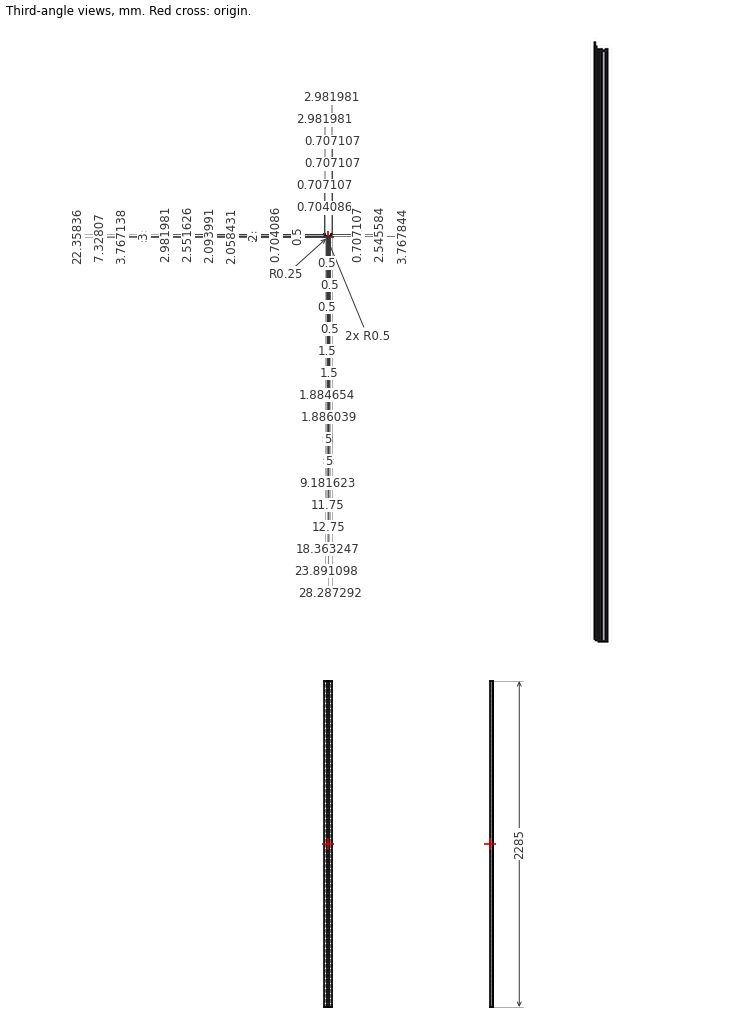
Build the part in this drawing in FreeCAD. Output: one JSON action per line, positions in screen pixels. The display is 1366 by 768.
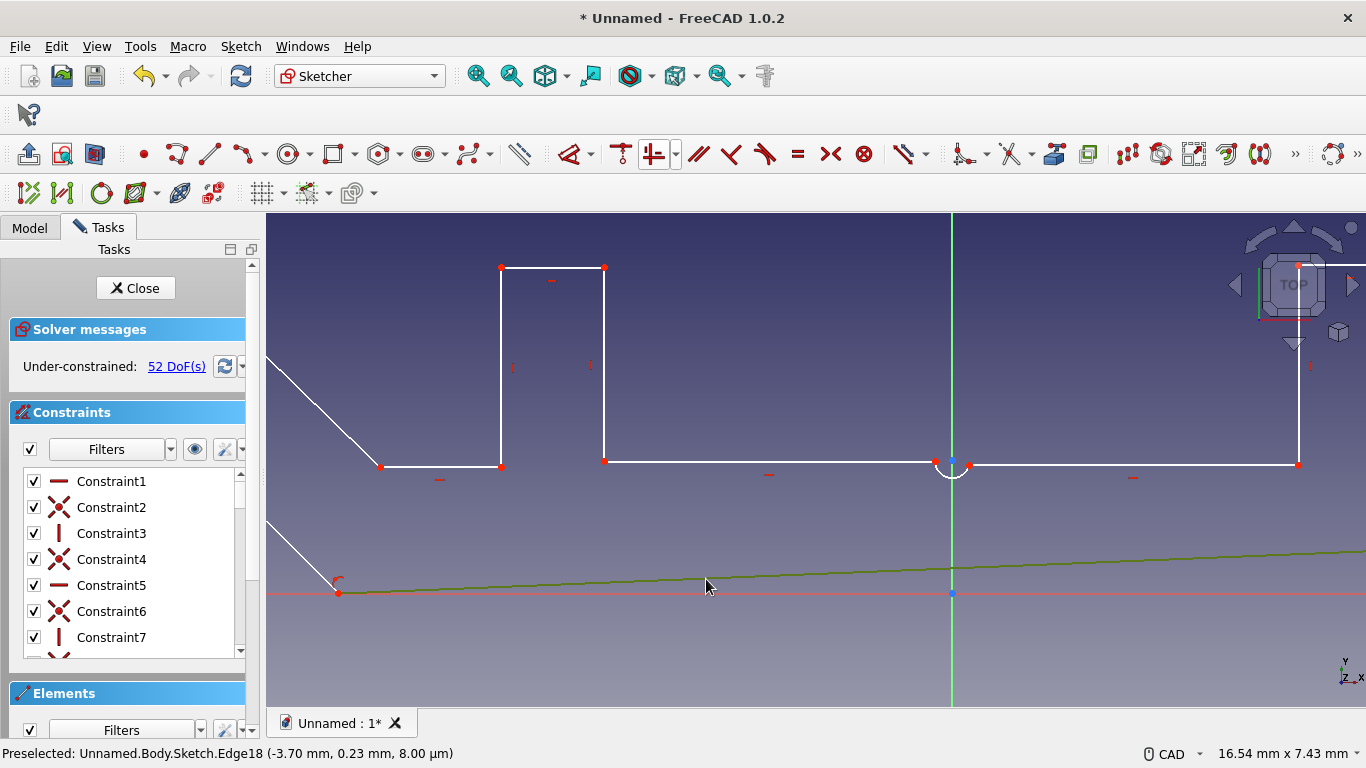
{"action": "key", "text": "h"}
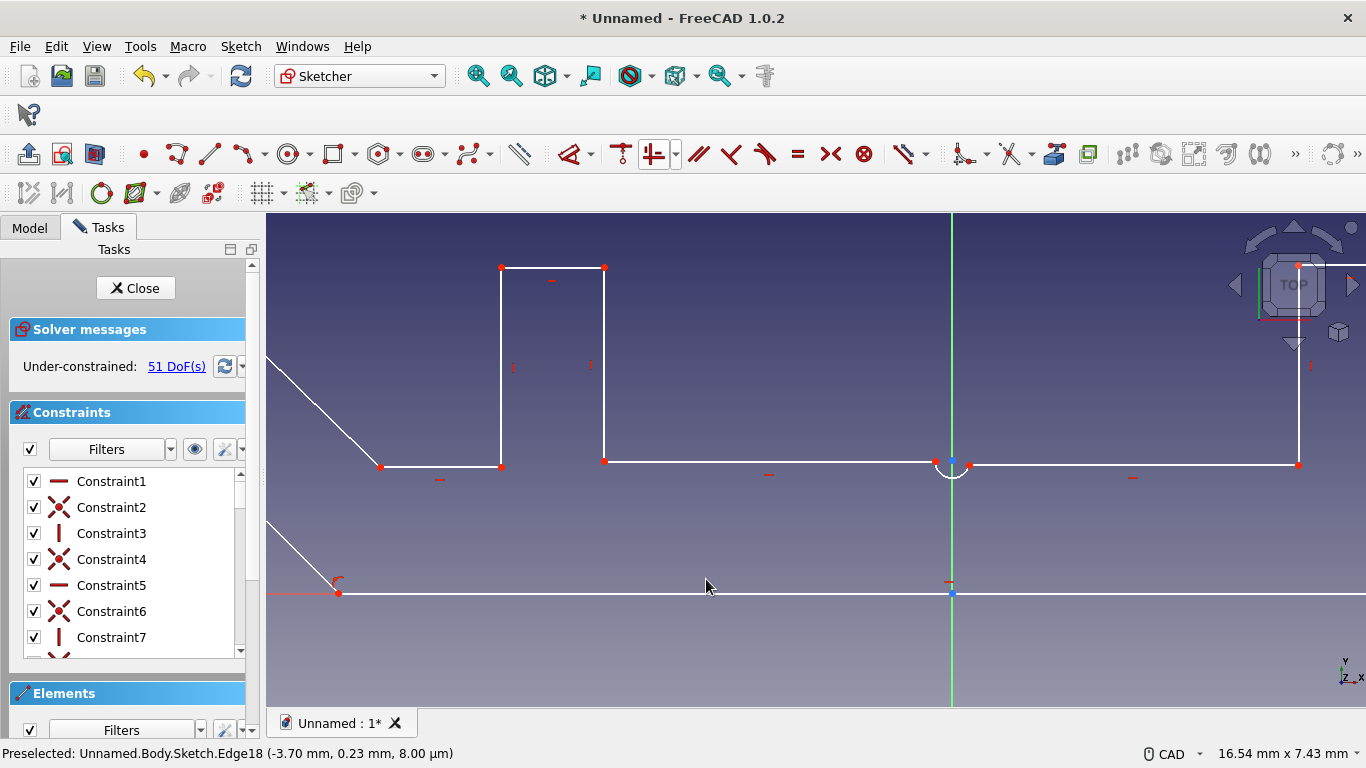
{"action": "scroll", "coordinate": [707, 581], "scroll_direction": "down", "scroll_amount": 9}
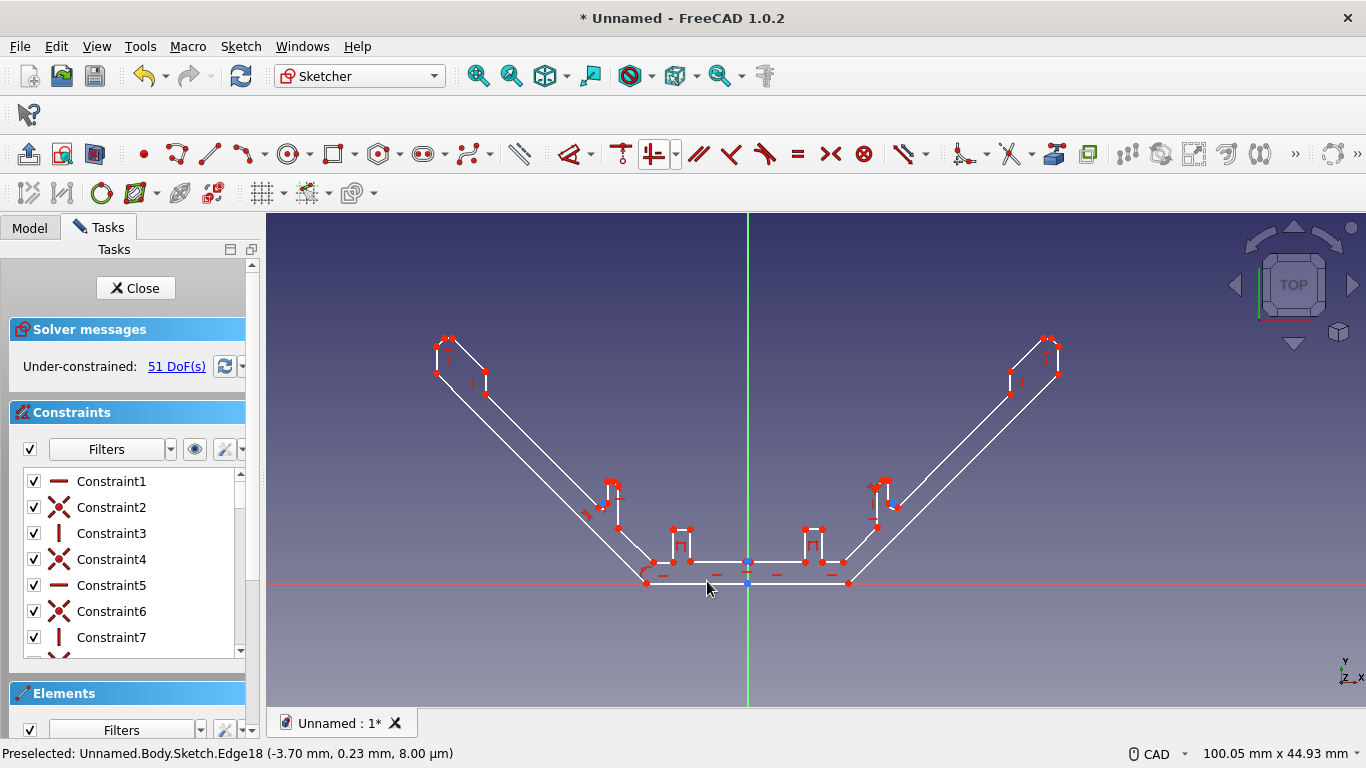
{"action": "scroll", "coordinate": [602, 509], "scroll_direction": "up", "scroll_amount": 7}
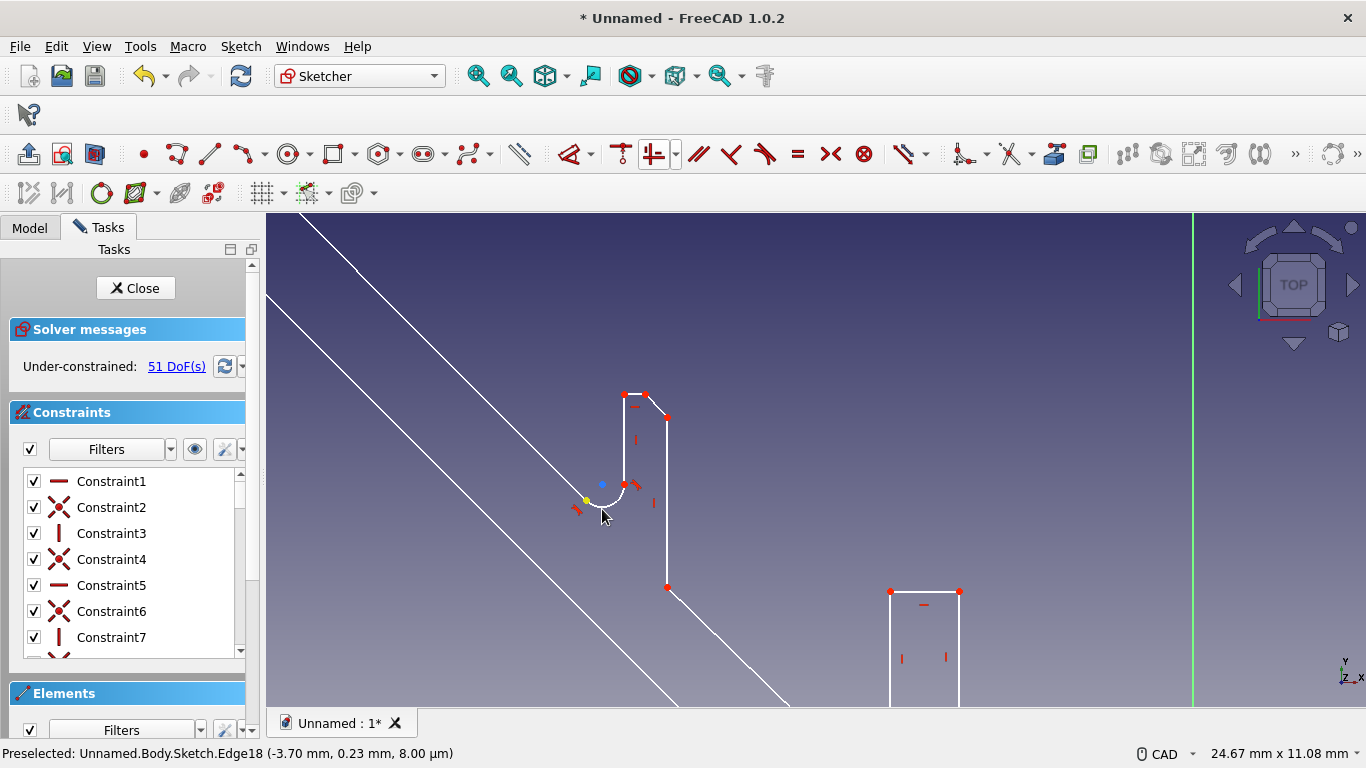
{"action": "left_click", "coordinate": [600, 507]}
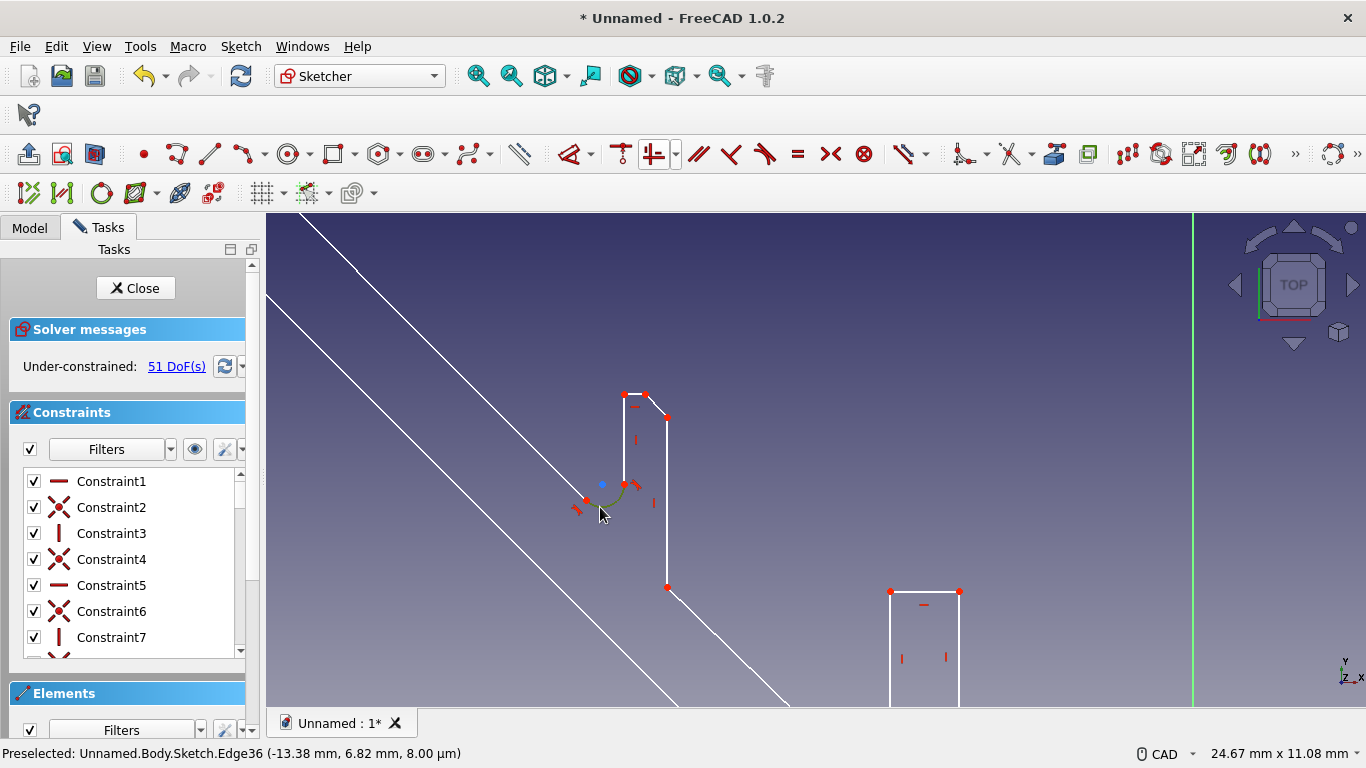
{"action": "scroll", "coordinate": [602, 509], "scroll_direction": "down", "scroll_amount": 7}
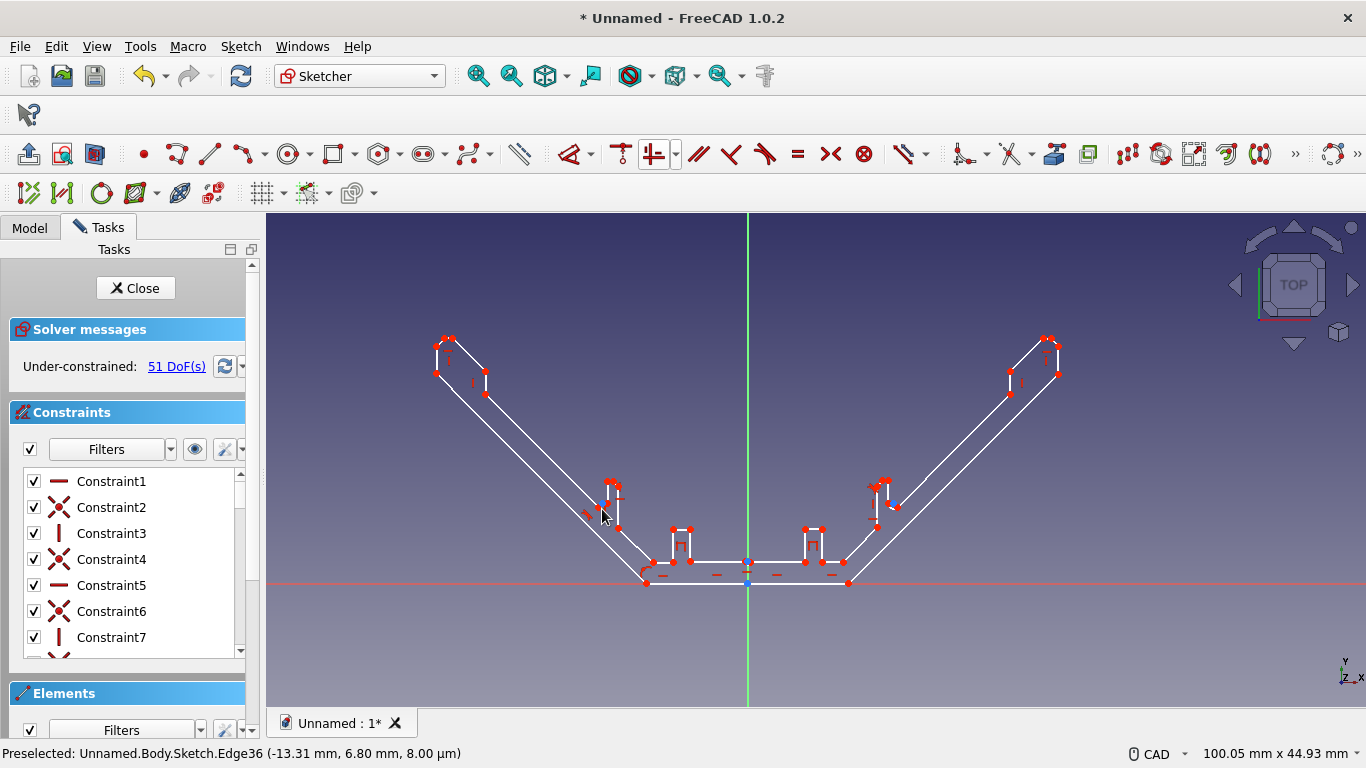
{"action": "scroll", "coordinate": [889, 507], "scroll_direction": "up", "scroll_amount": 7}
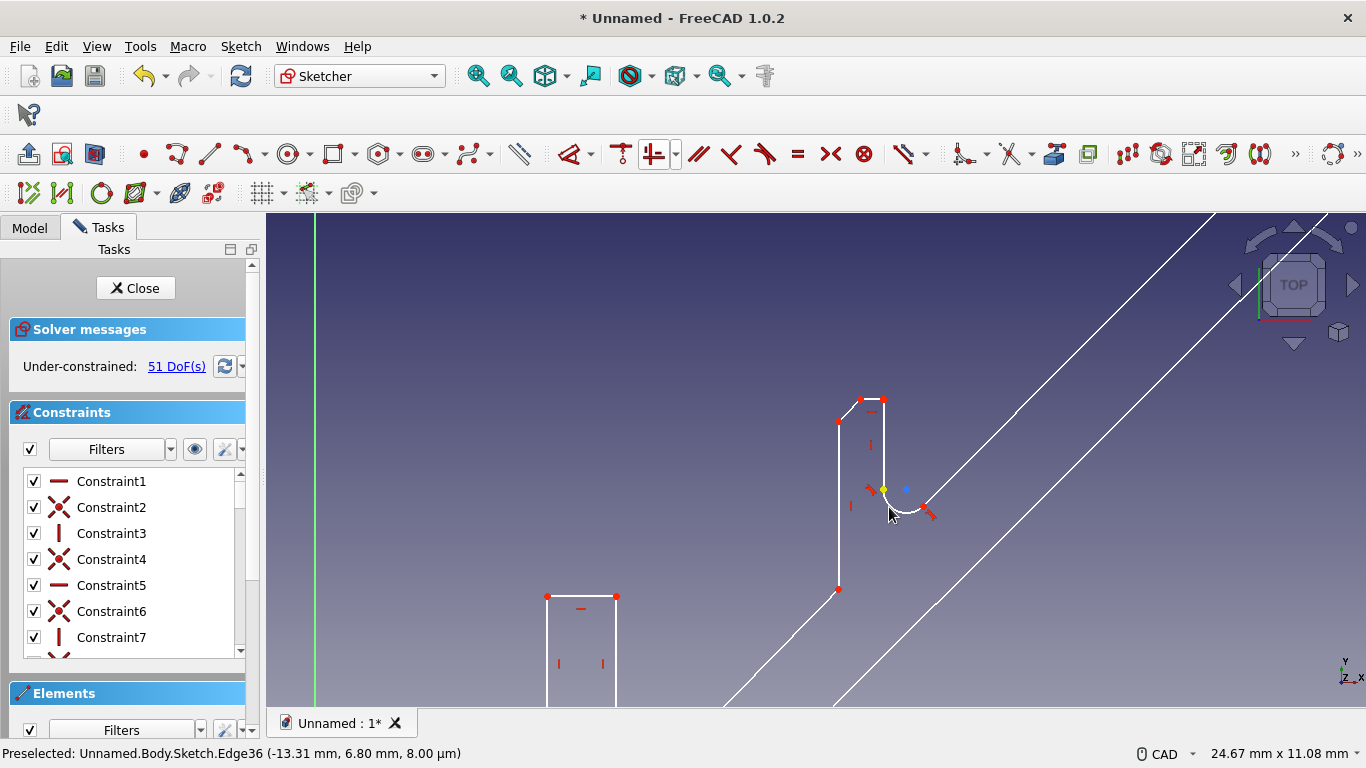
{"action": "left_click", "coordinate": [889, 505]}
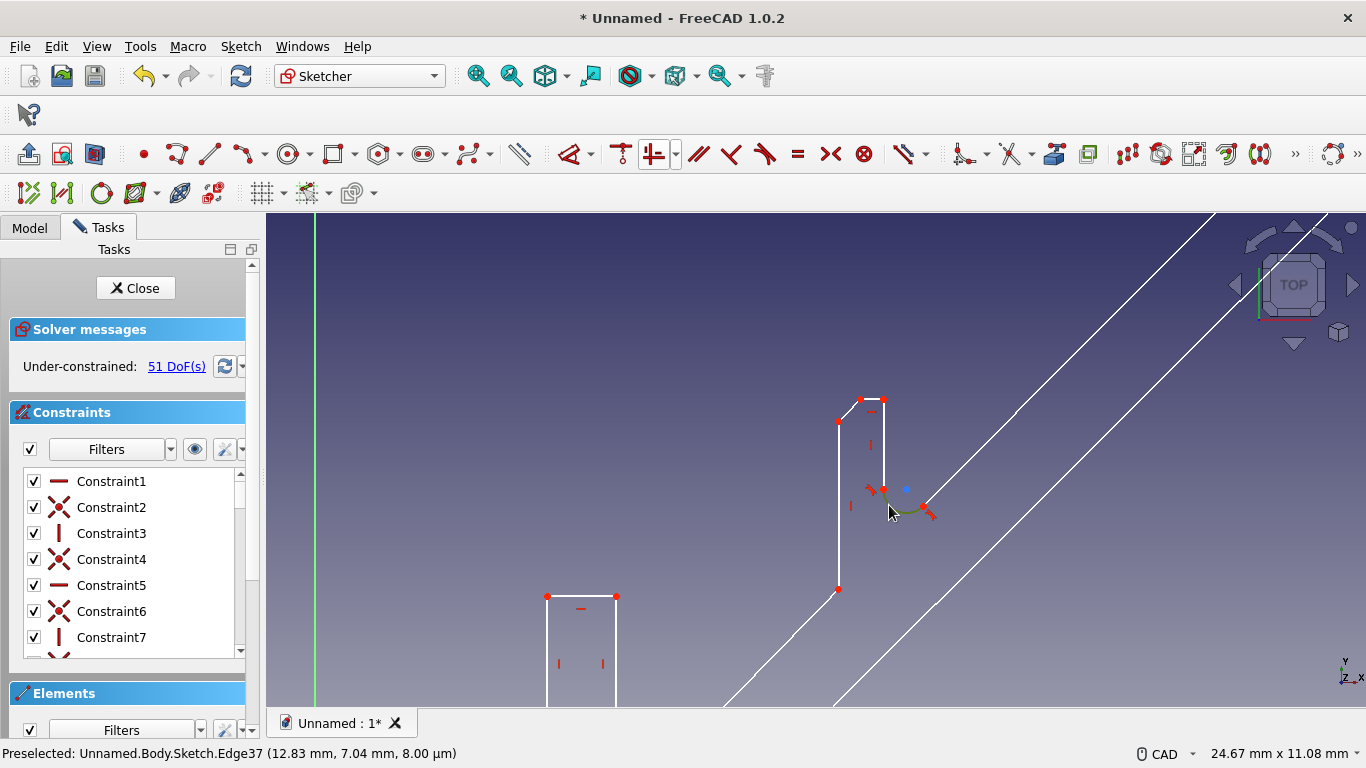
{"action": "left_click", "coordinate": [798, 154]}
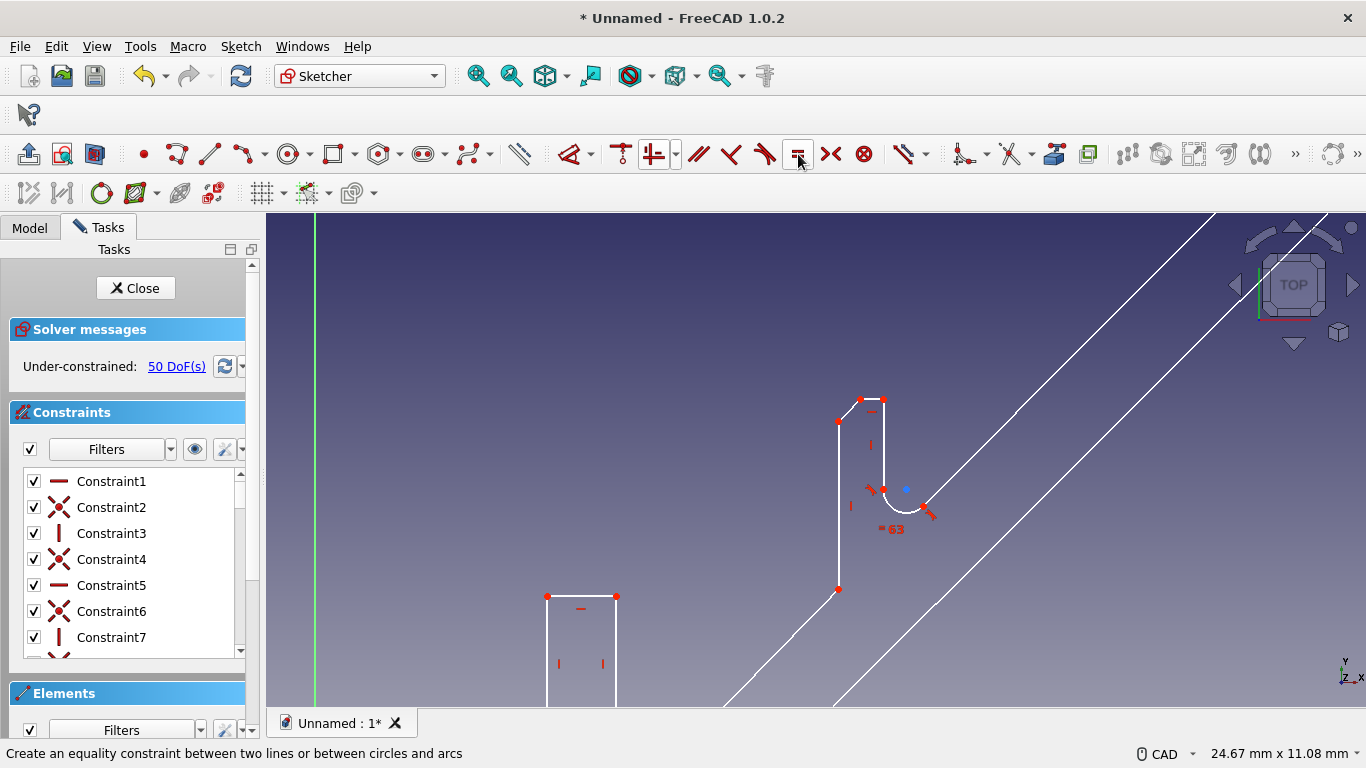
{"action": "scroll", "coordinate": [889, 507], "scroll_direction": "down", "scroll_amount": 7}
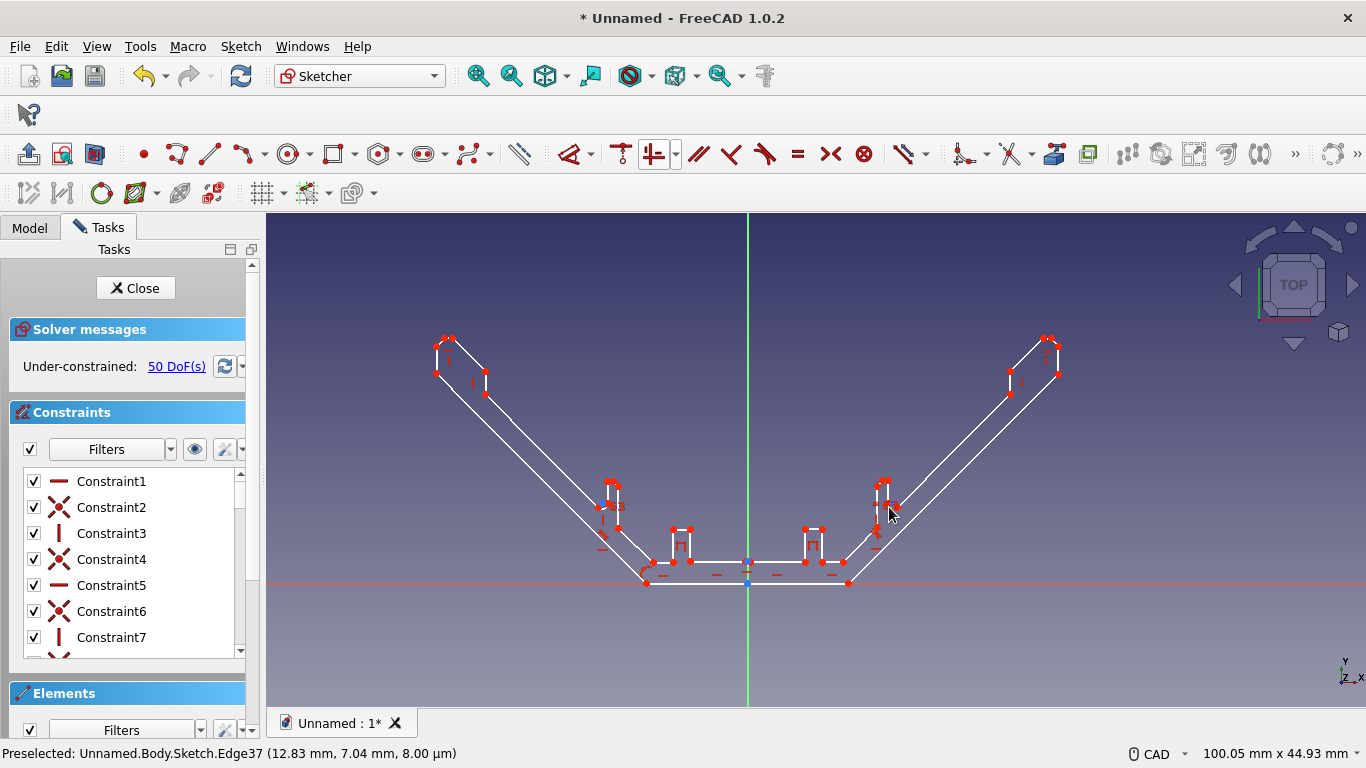
{"action": "scroll", "coordinate": [748, 562], "scroll_direction": "up", "scroll_amount": 8}